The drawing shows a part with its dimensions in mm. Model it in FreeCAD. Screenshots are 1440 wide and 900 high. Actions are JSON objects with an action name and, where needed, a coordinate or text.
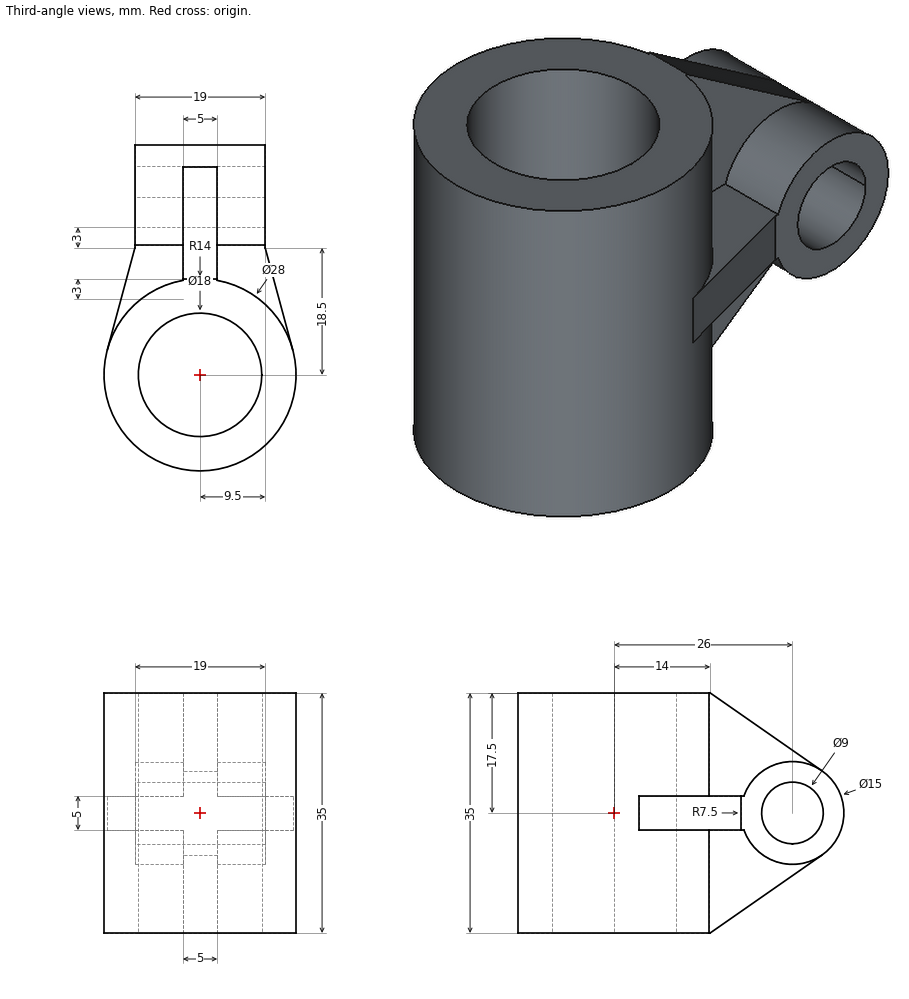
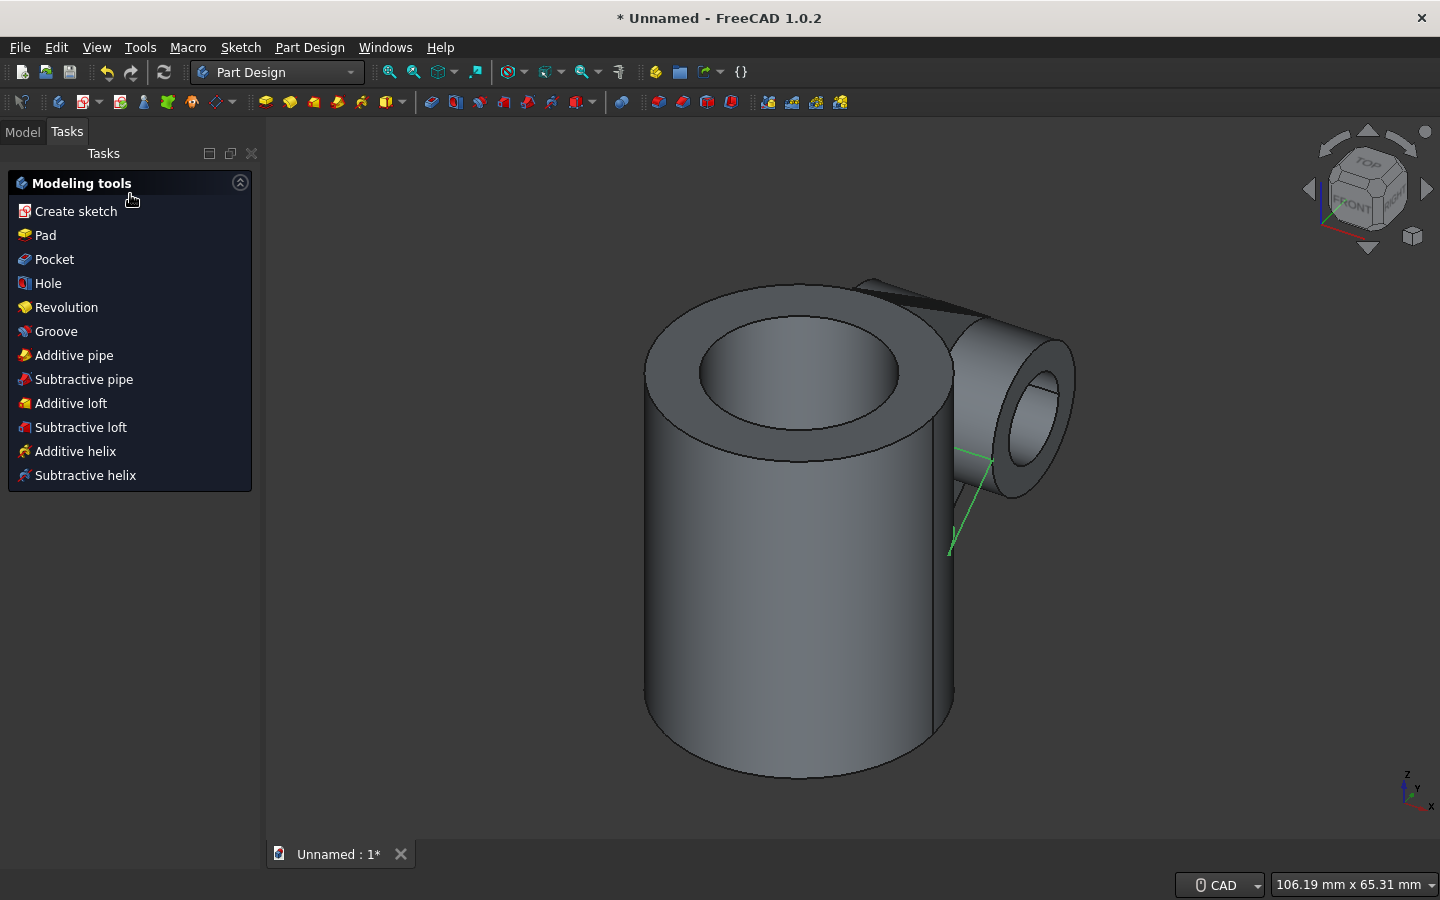
{"action": "left_click", "coordinate": [266, 102]}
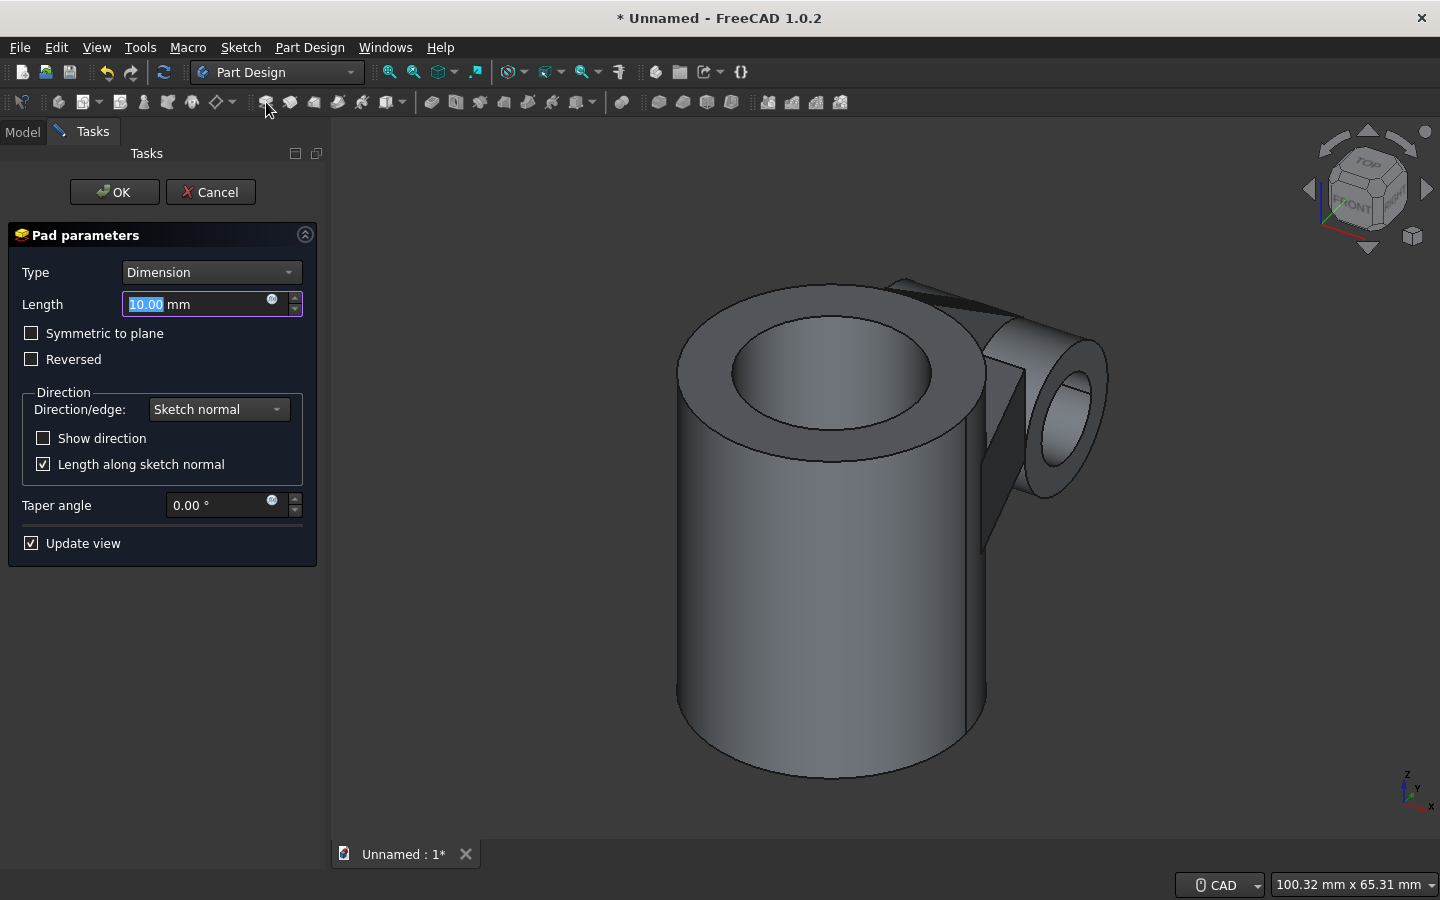
{"action": "type", "text": "5"}
{"action": "key", "text": "Tab"}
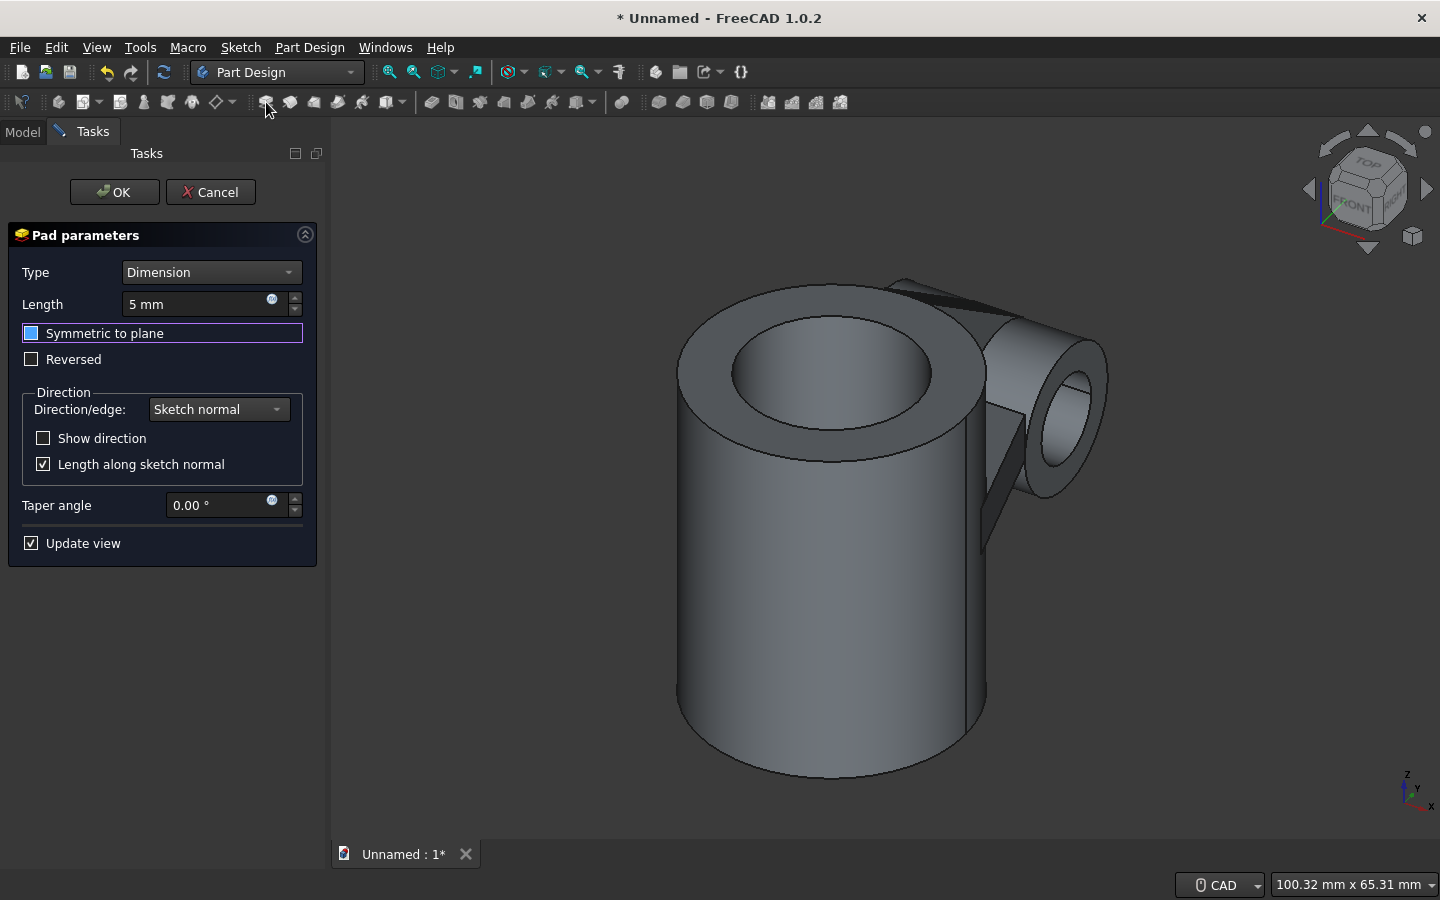
{"action": "left_click", "coordinate": [30, 333]}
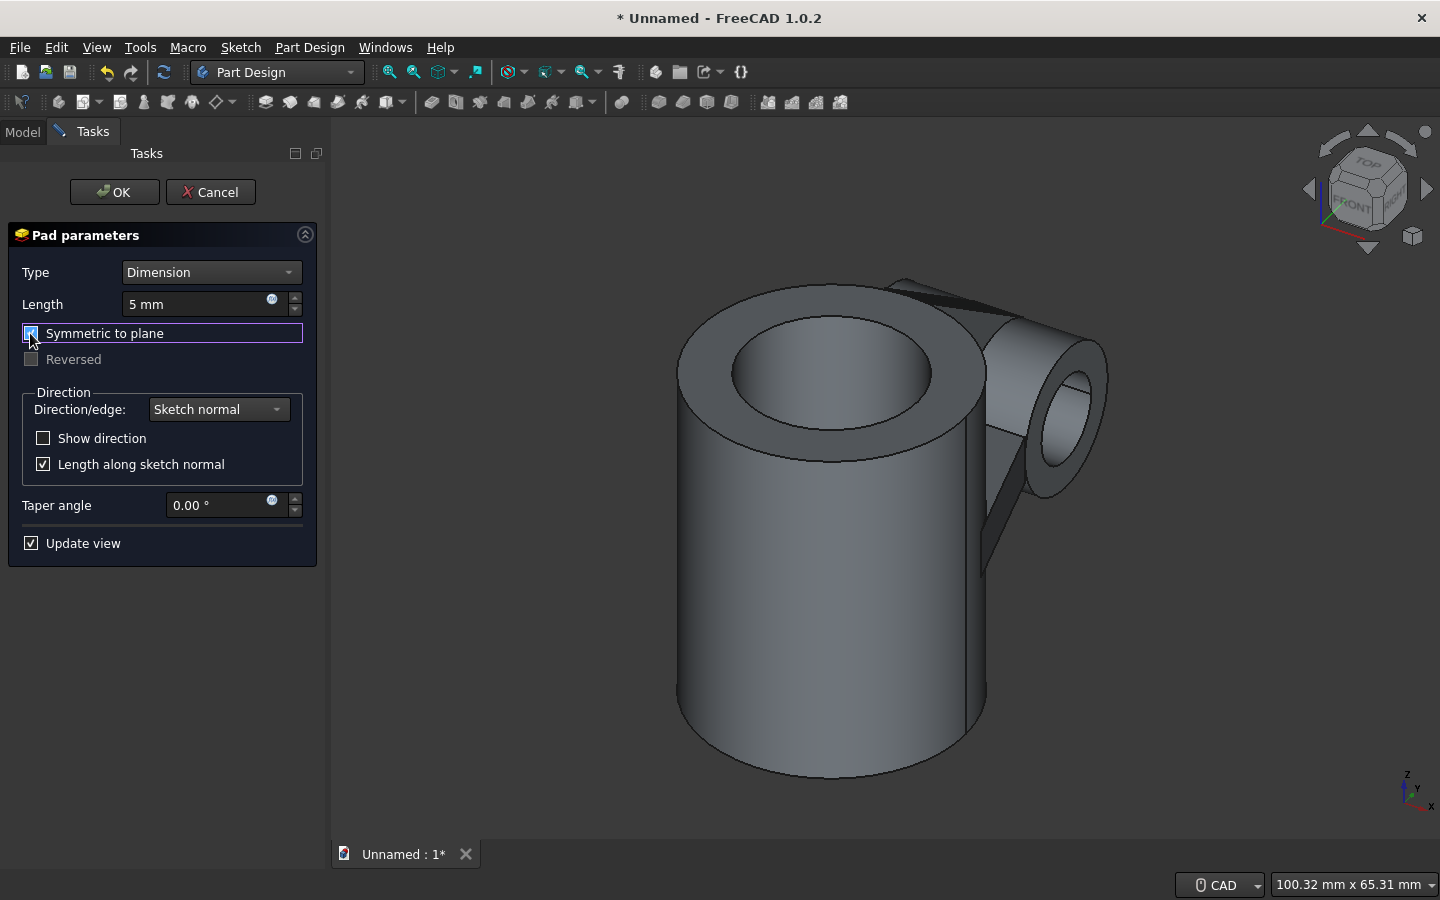
{"action": "left_click", "coordinate": [115, 192]}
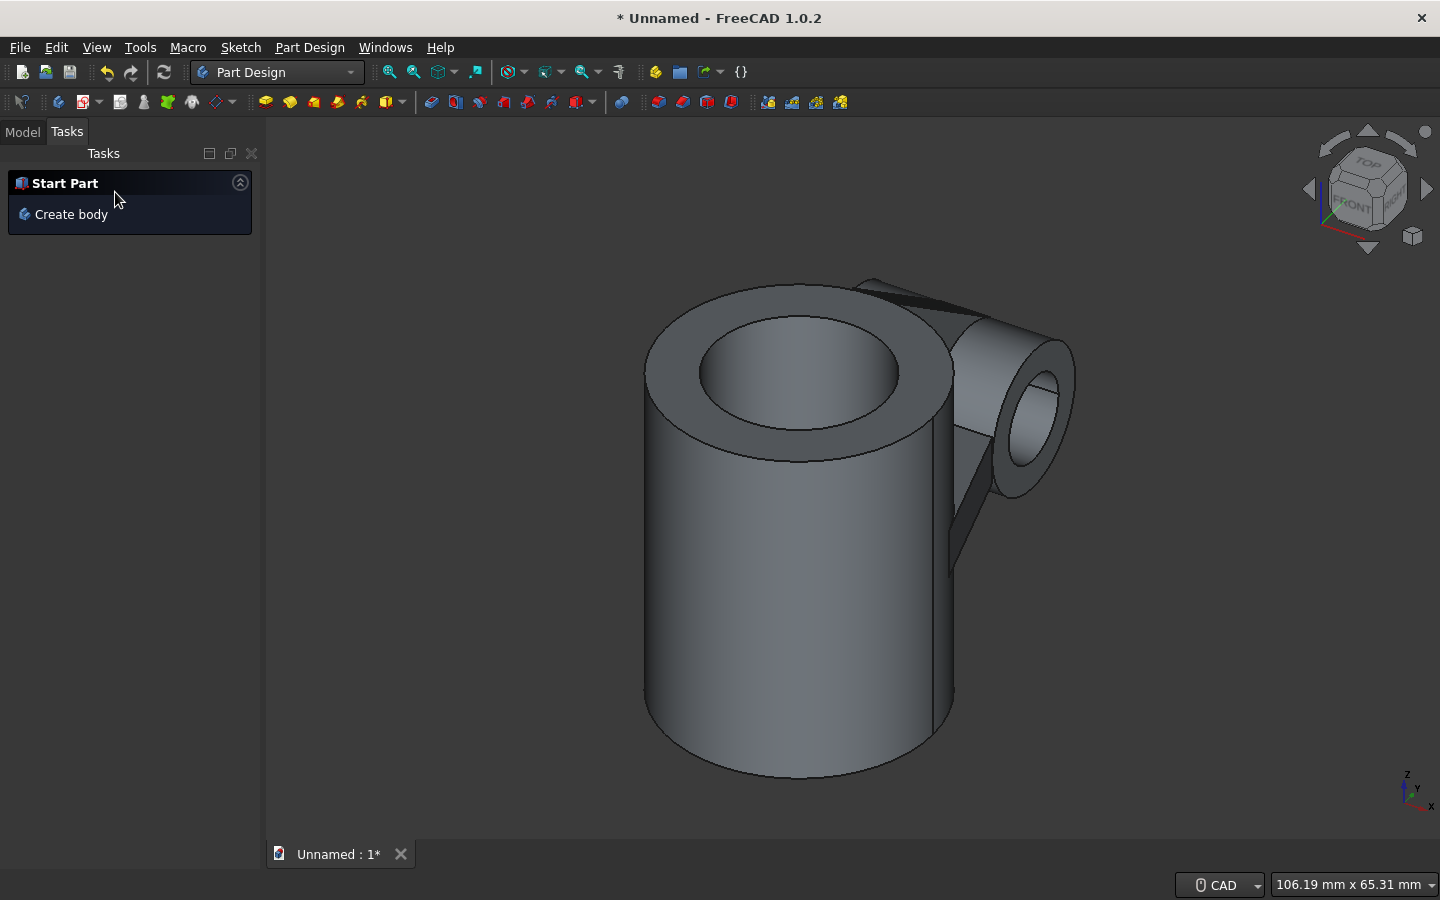
{"action": "key", "text": "v f"}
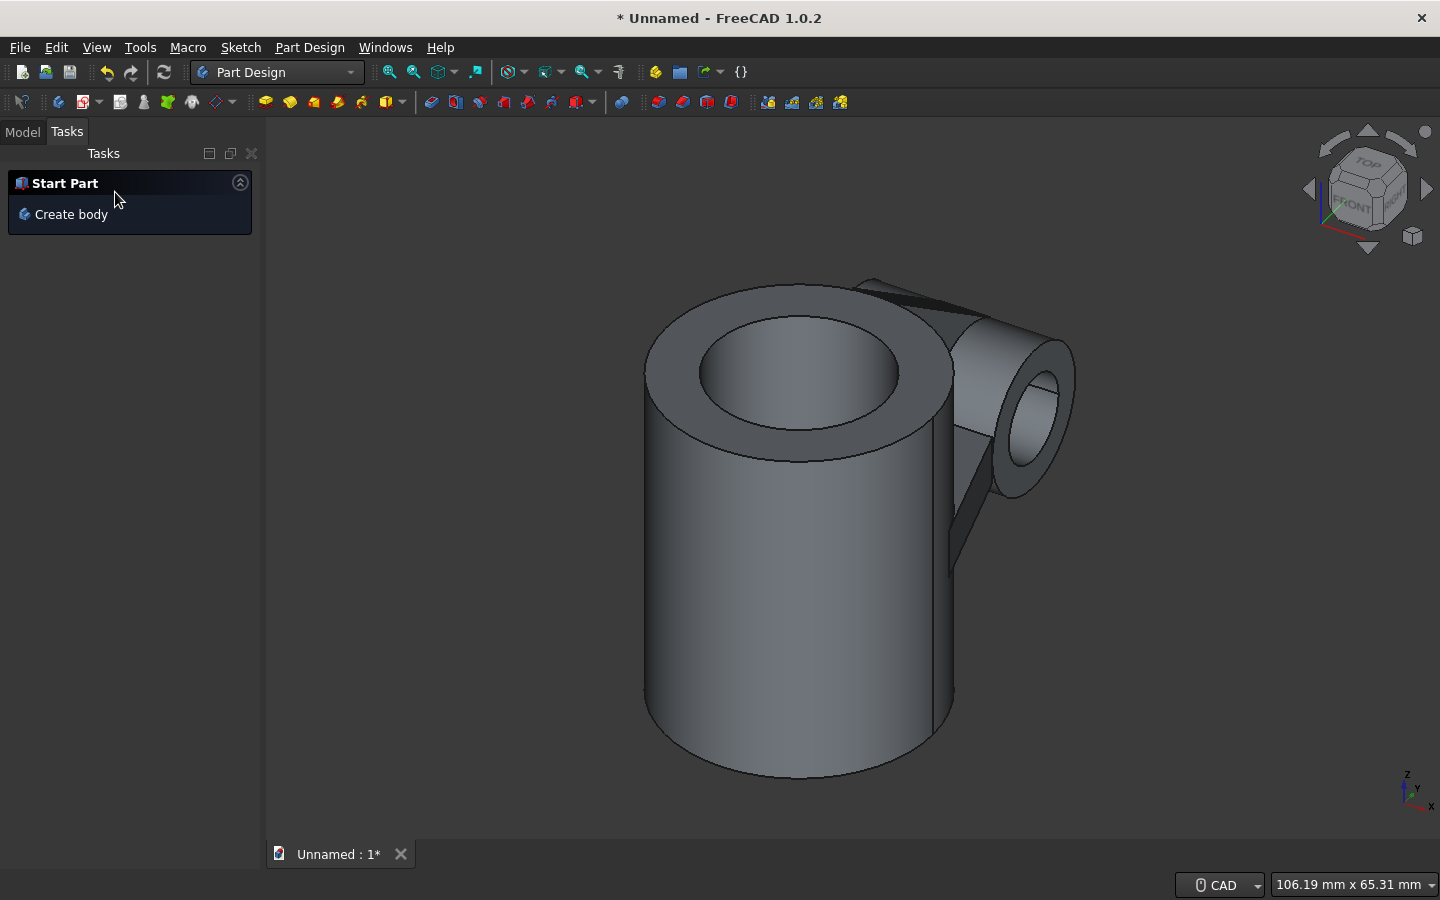
{"action": "left_click", "coordinate": [23, 131]}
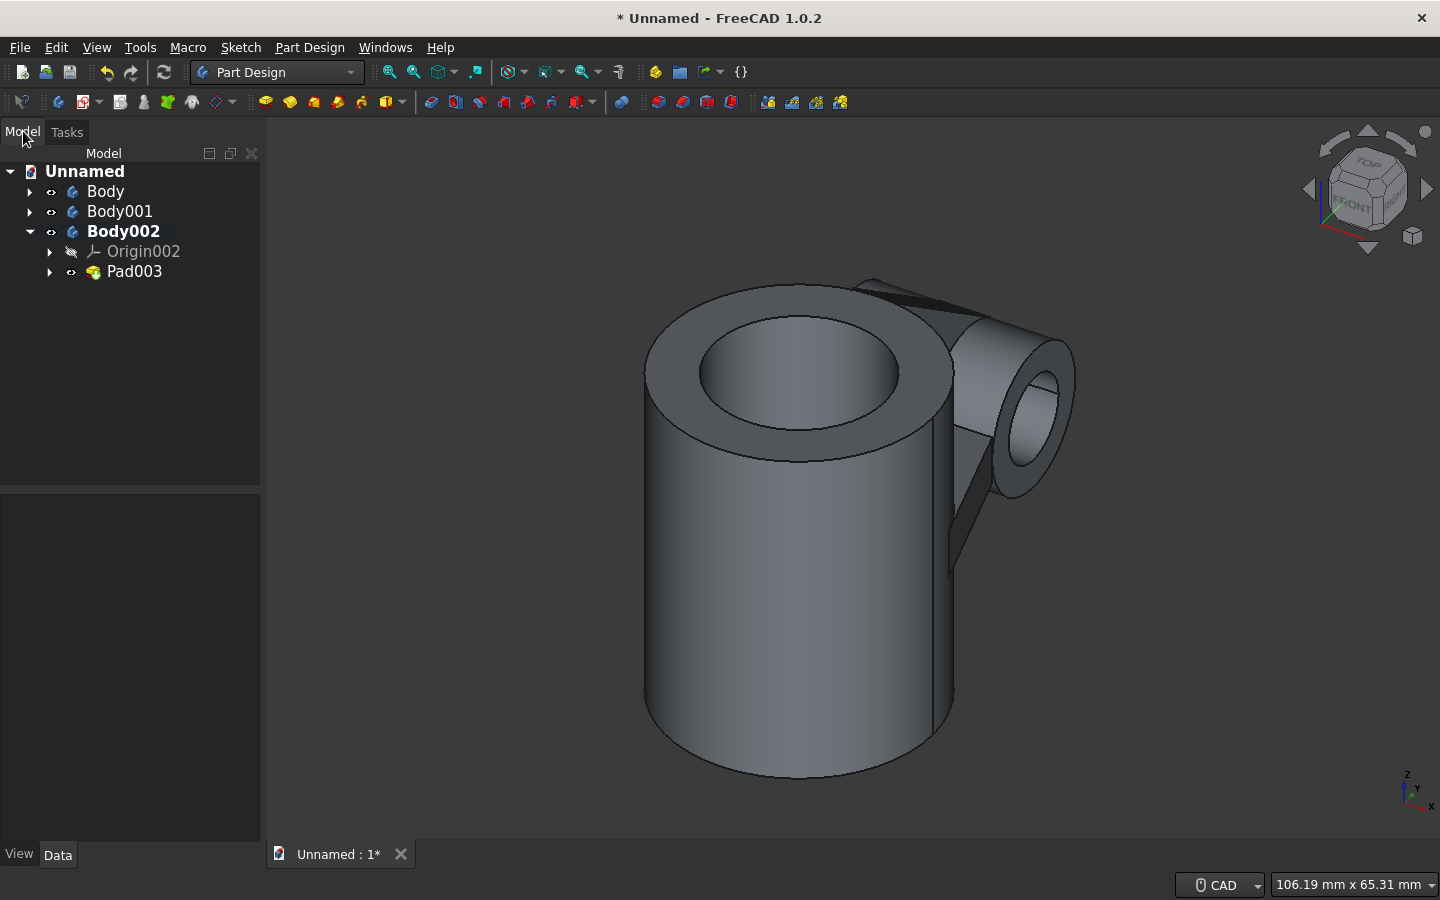
{"action": "double_click", "coordinate": [96, 212]}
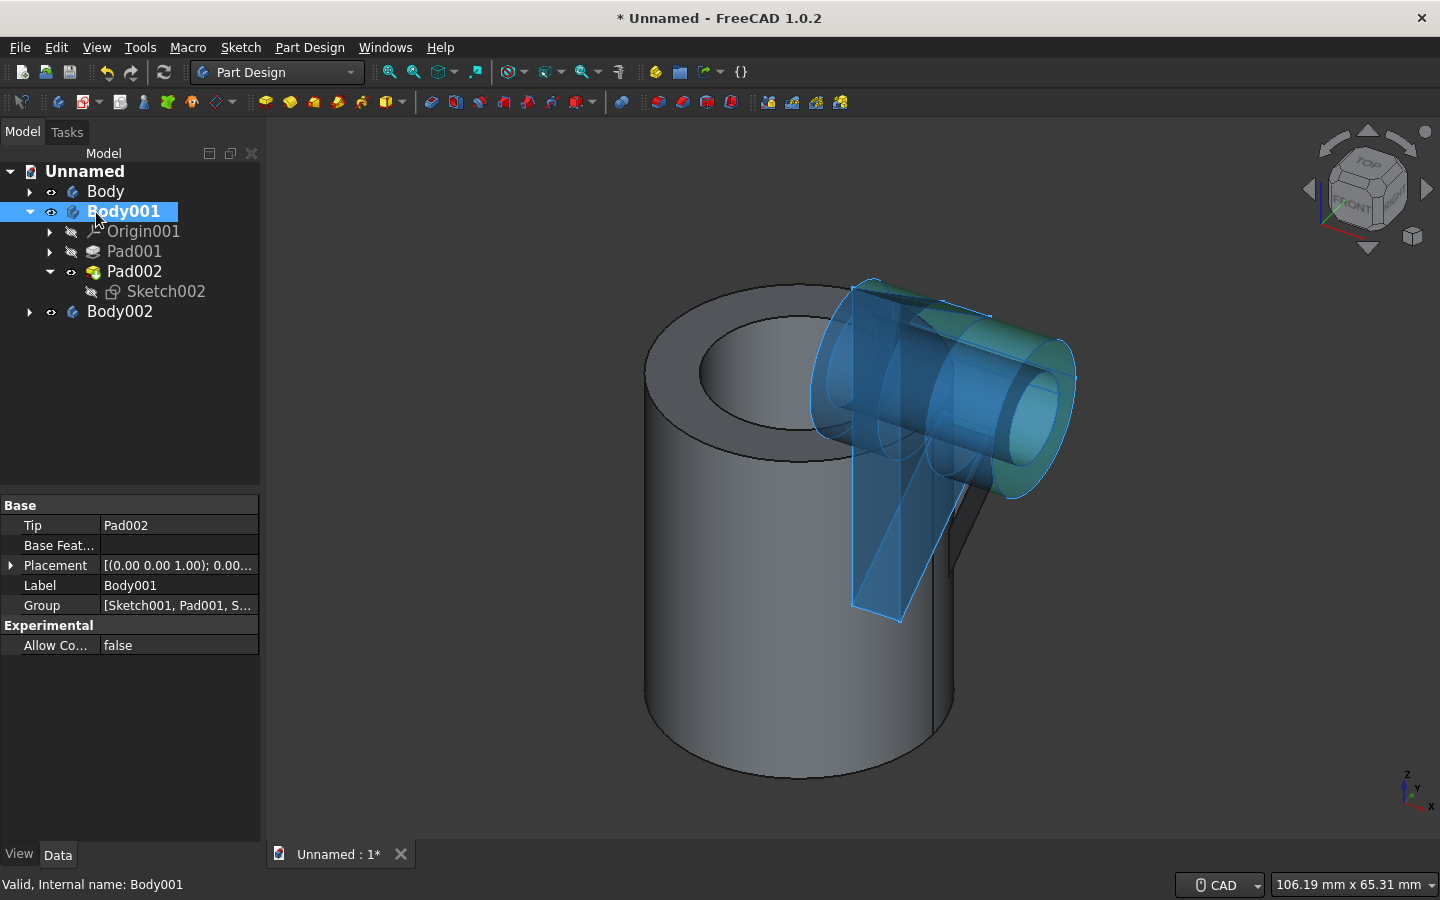
{"action": "left_click", "coordinate": [96, 312]}